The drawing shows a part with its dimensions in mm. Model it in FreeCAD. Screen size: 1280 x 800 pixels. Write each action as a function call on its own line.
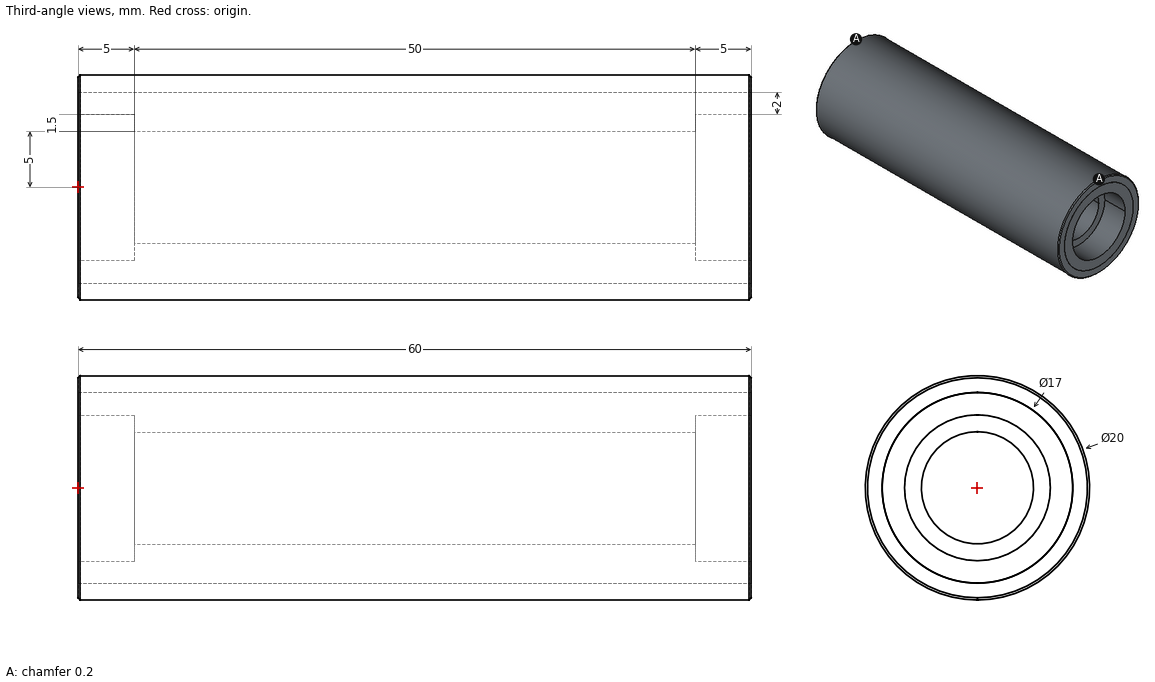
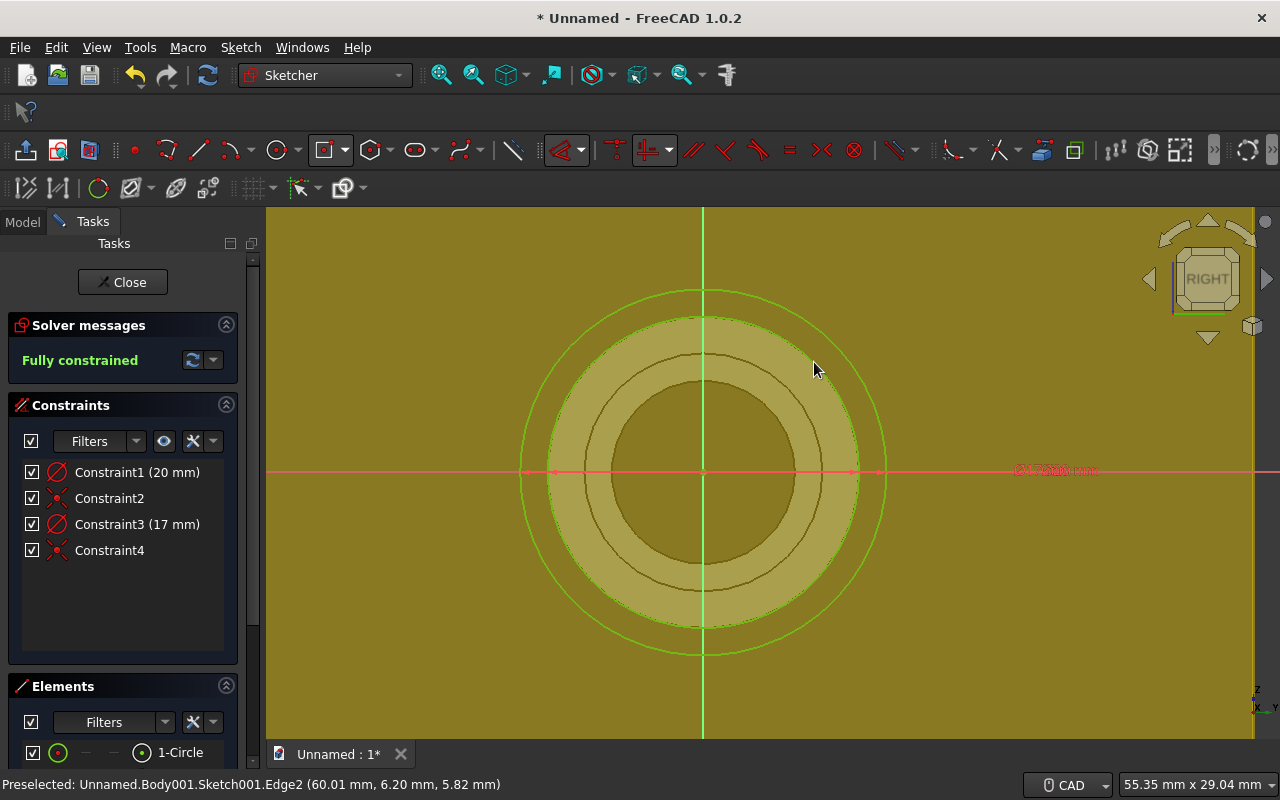
click(123, 282)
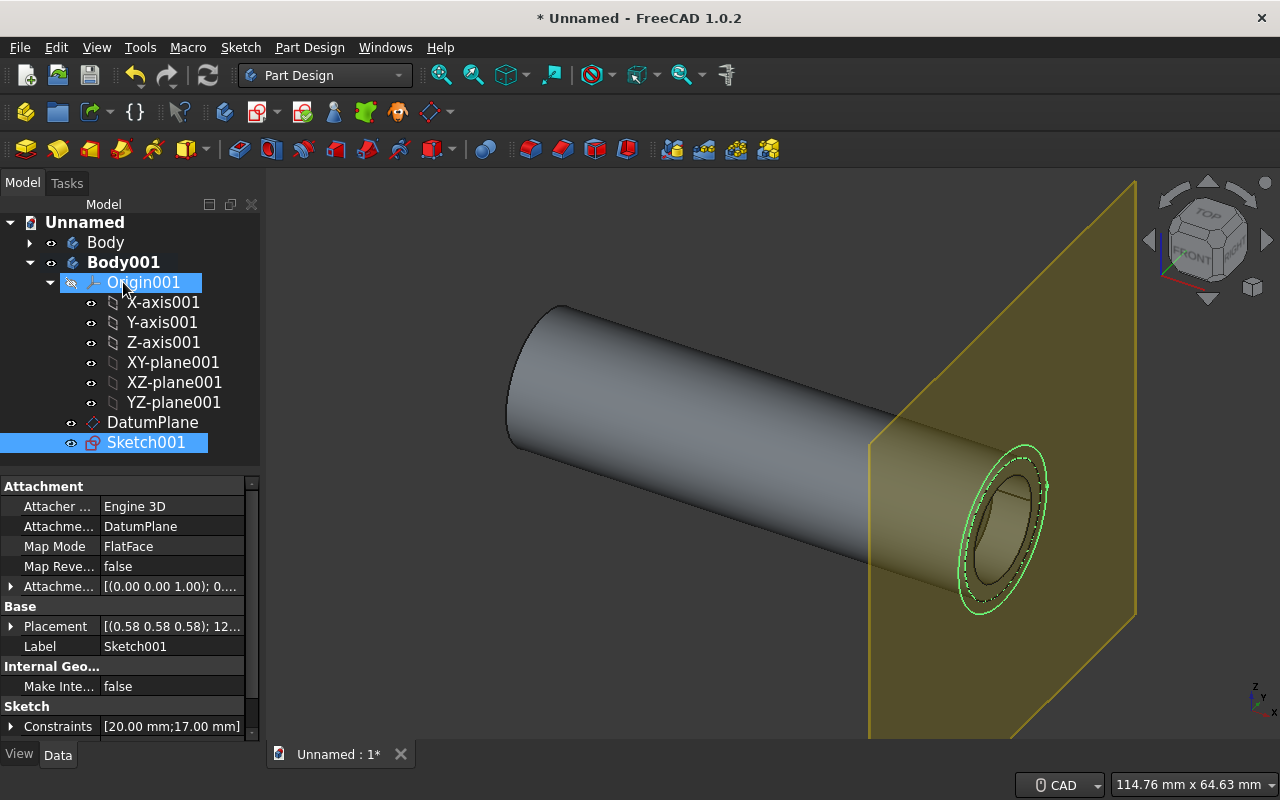
click(26, 150)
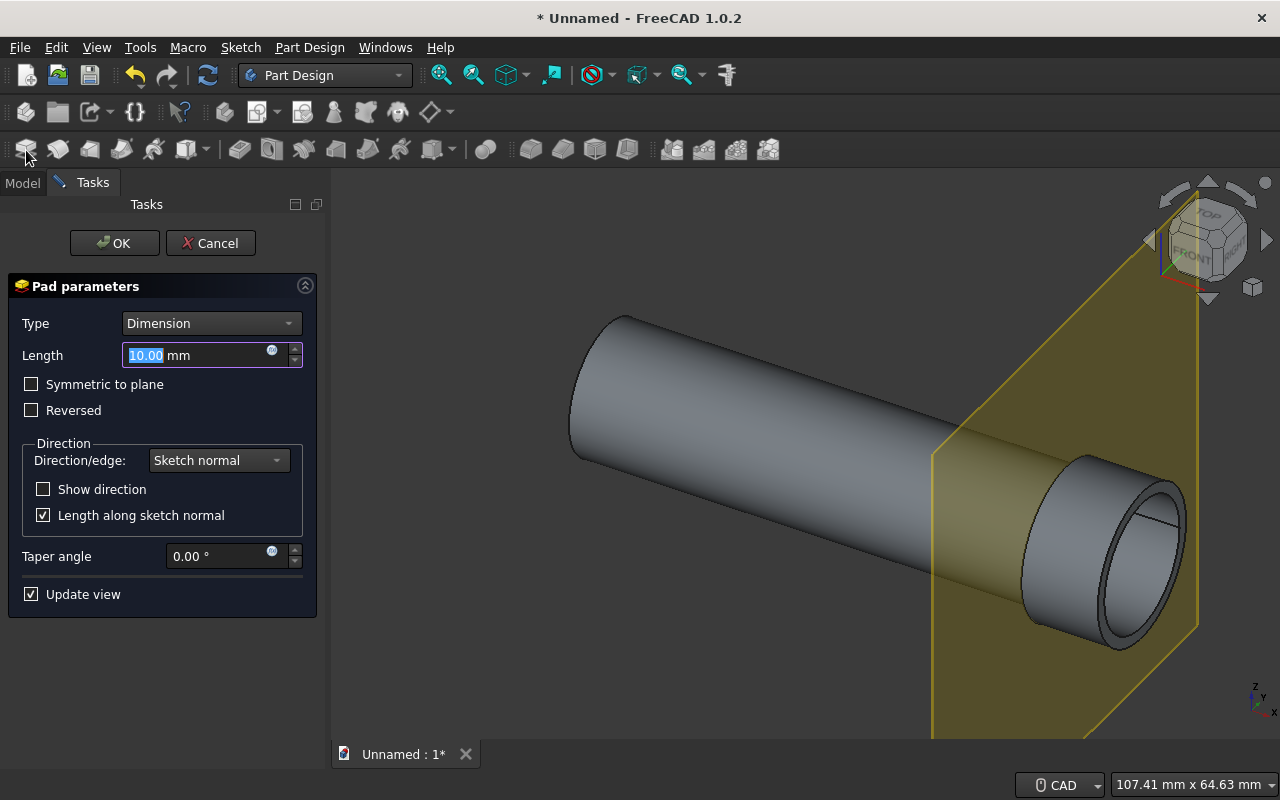
text(60)
key(Tab)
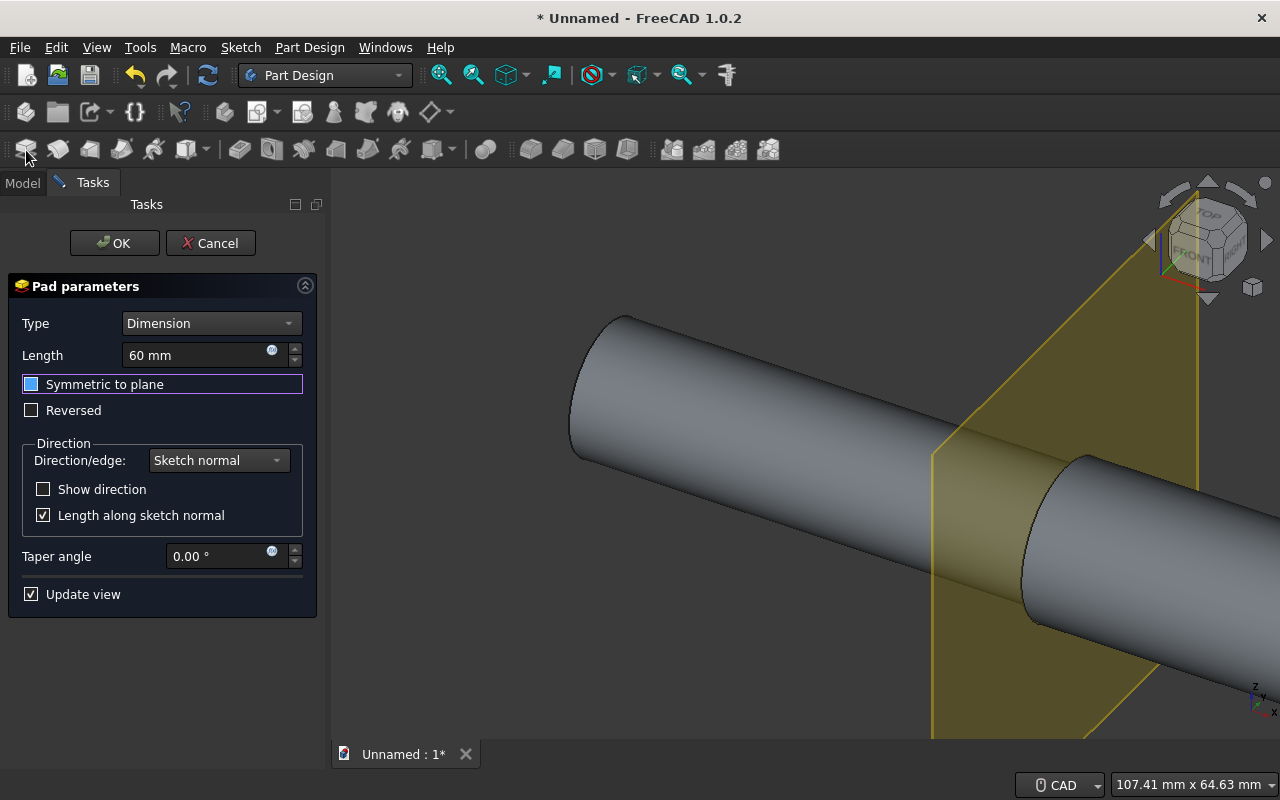
click(30, 410)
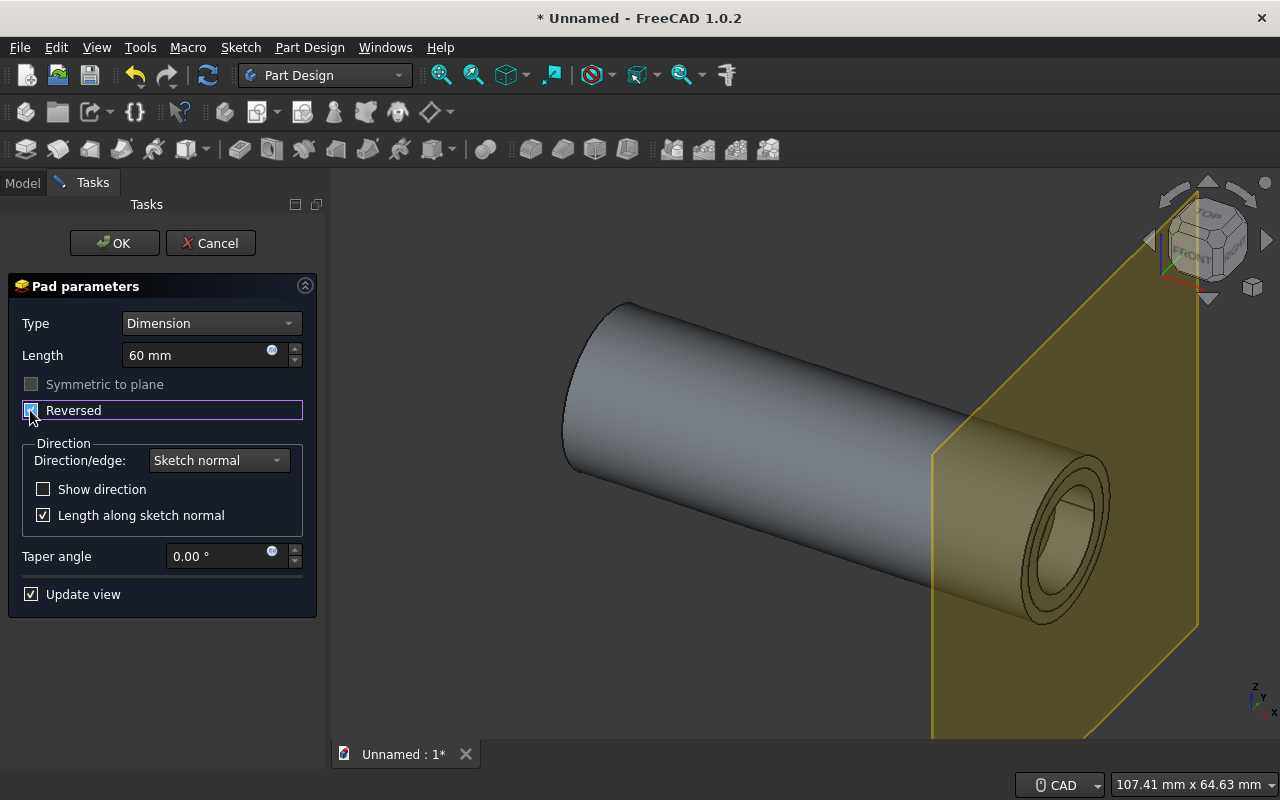
click(115, 243)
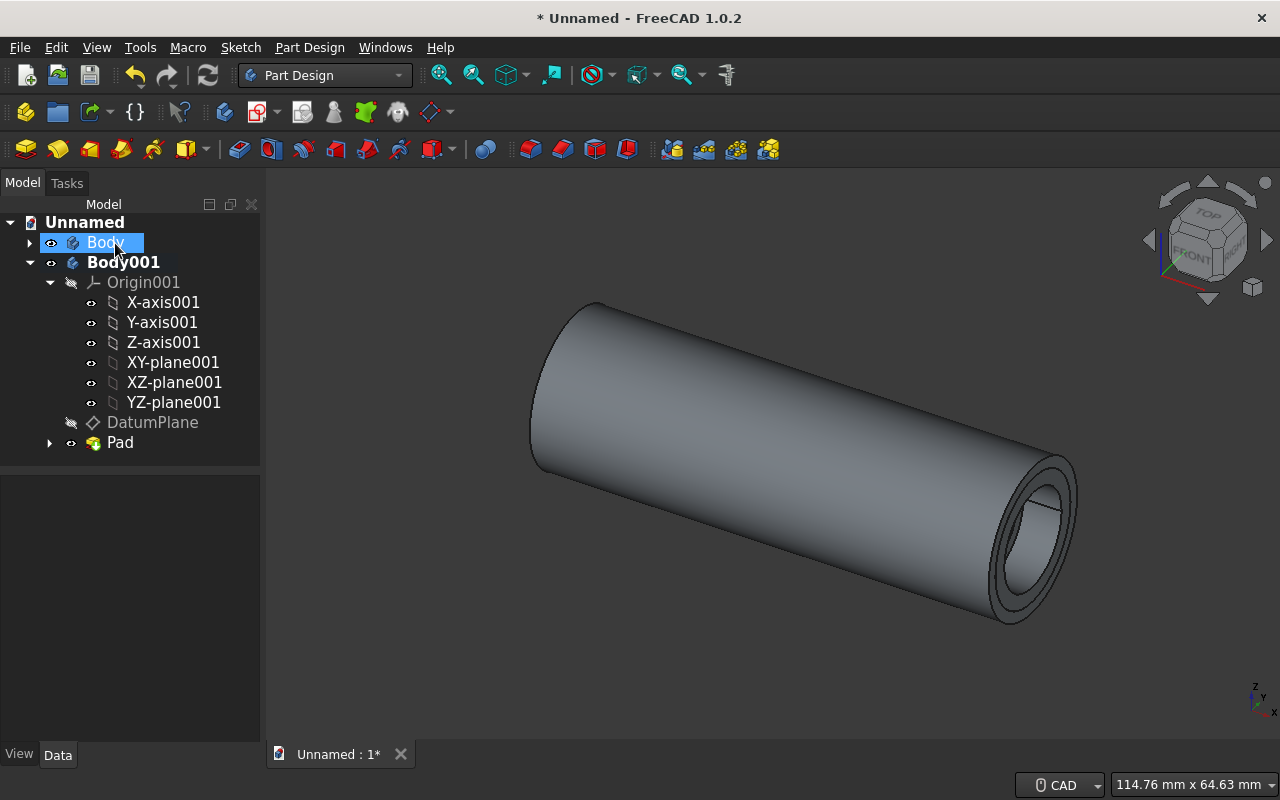
click(989, 583)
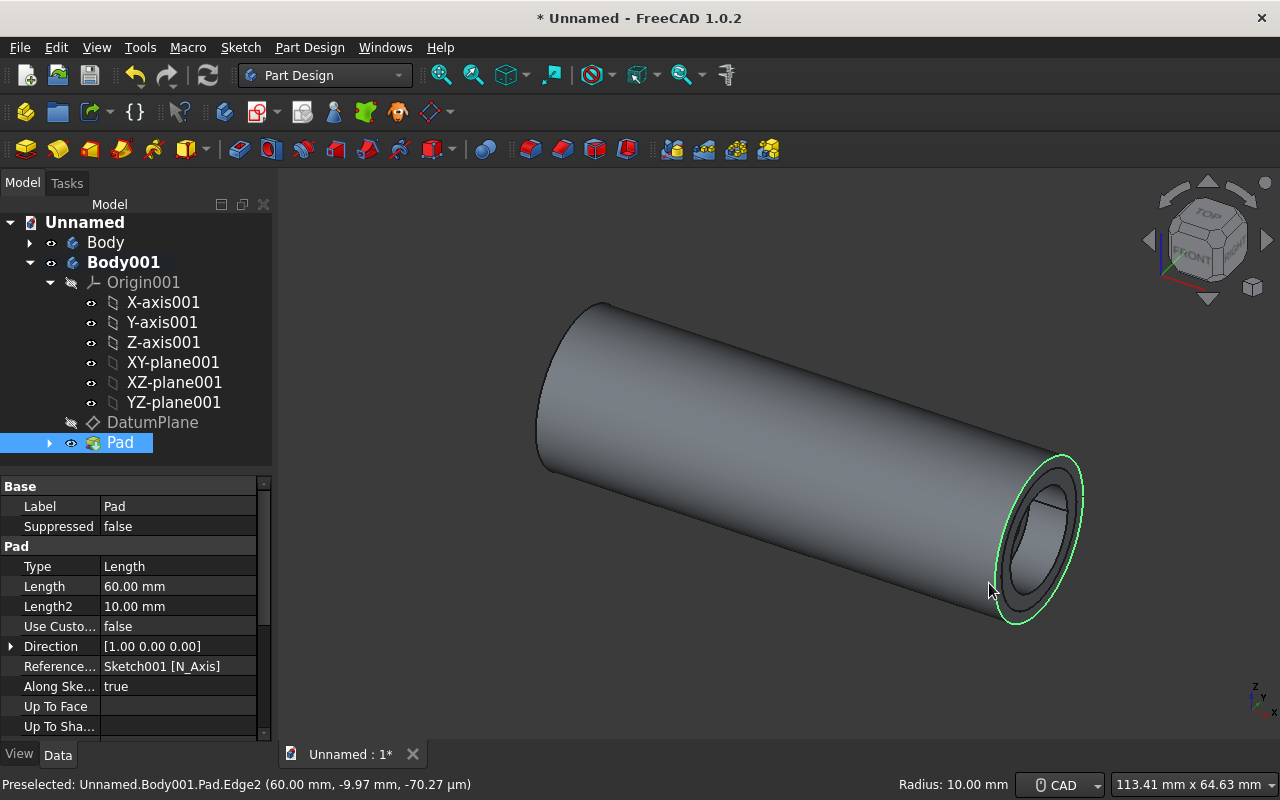
click(544, 465, ctrl)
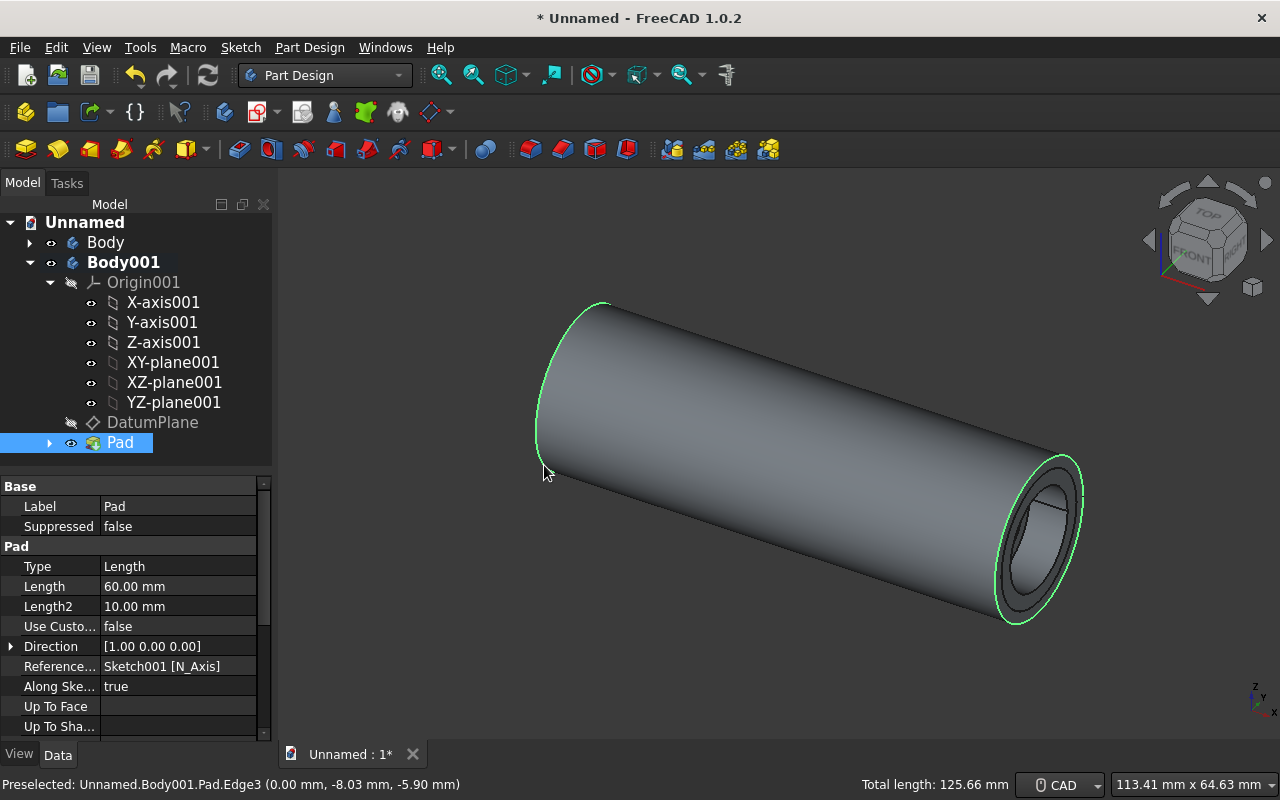
click(564, 150)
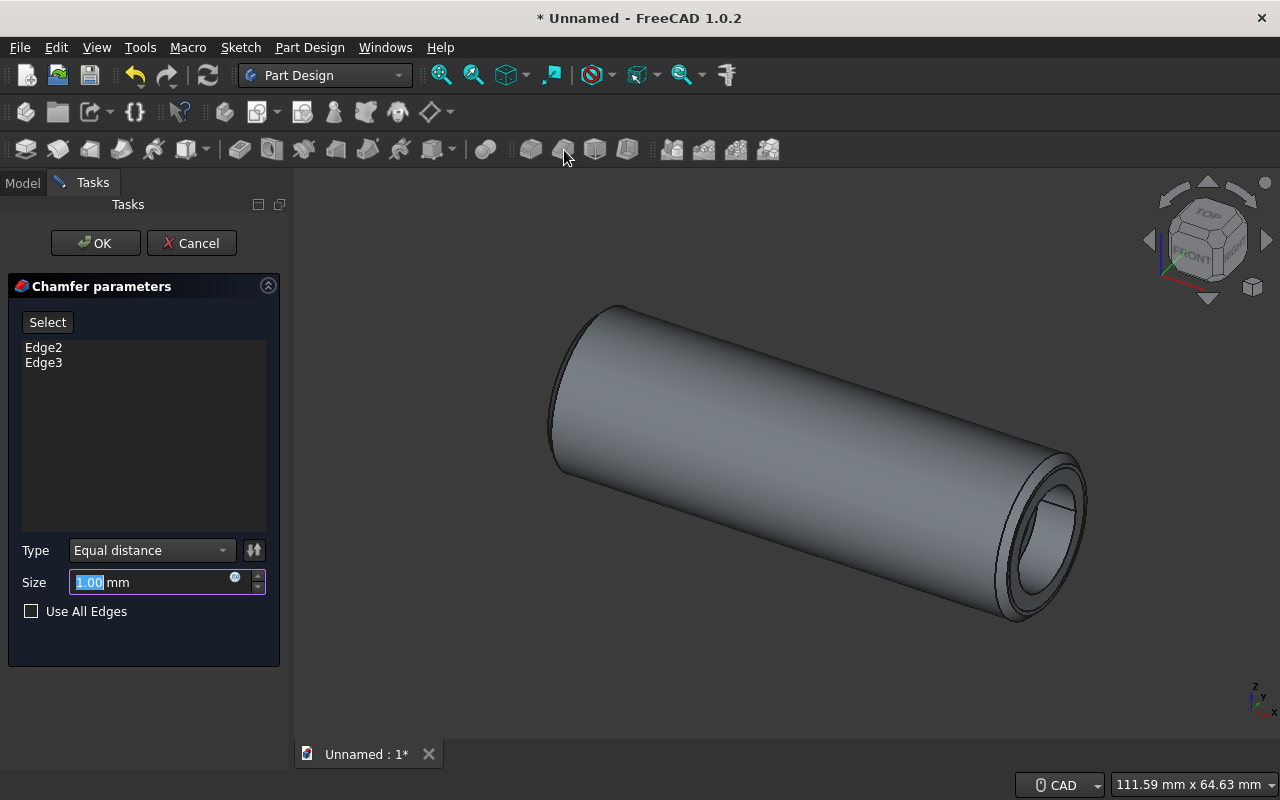
text(0.2)
key(Tab)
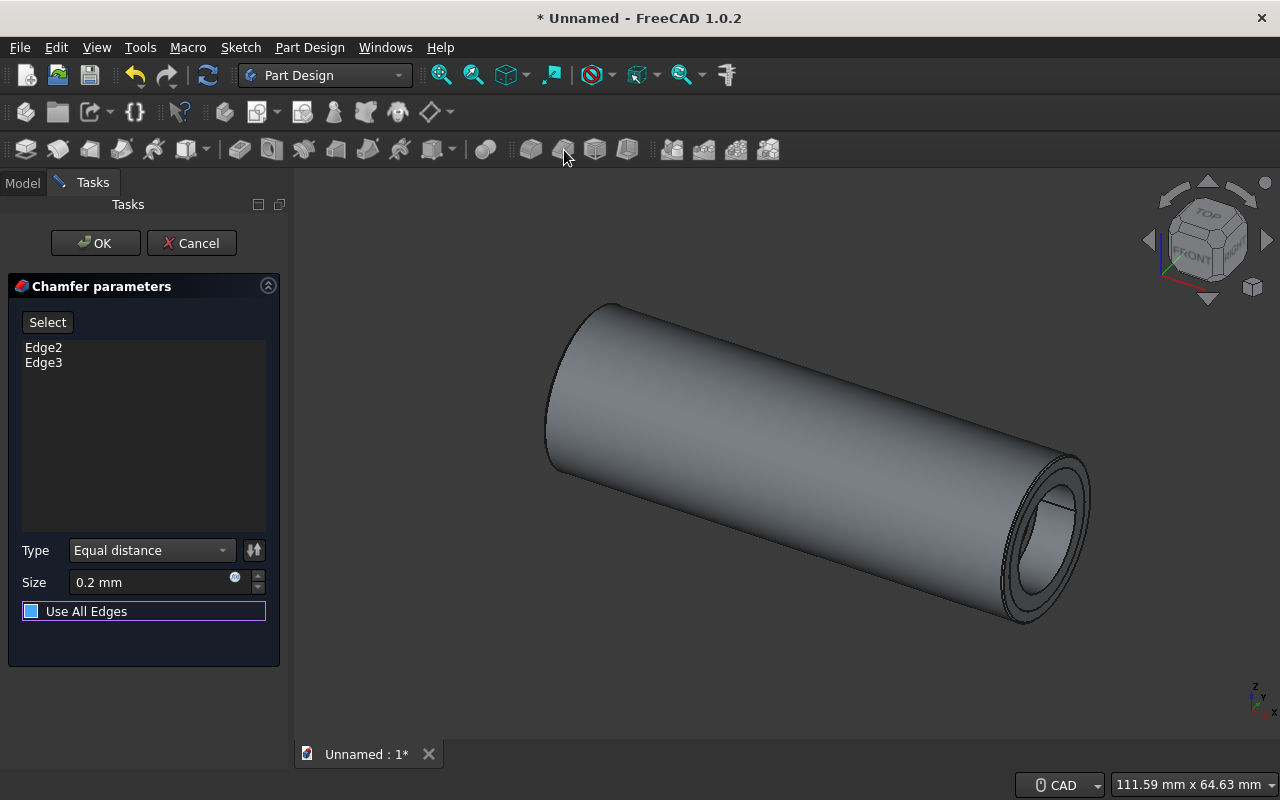
click(96, 243)